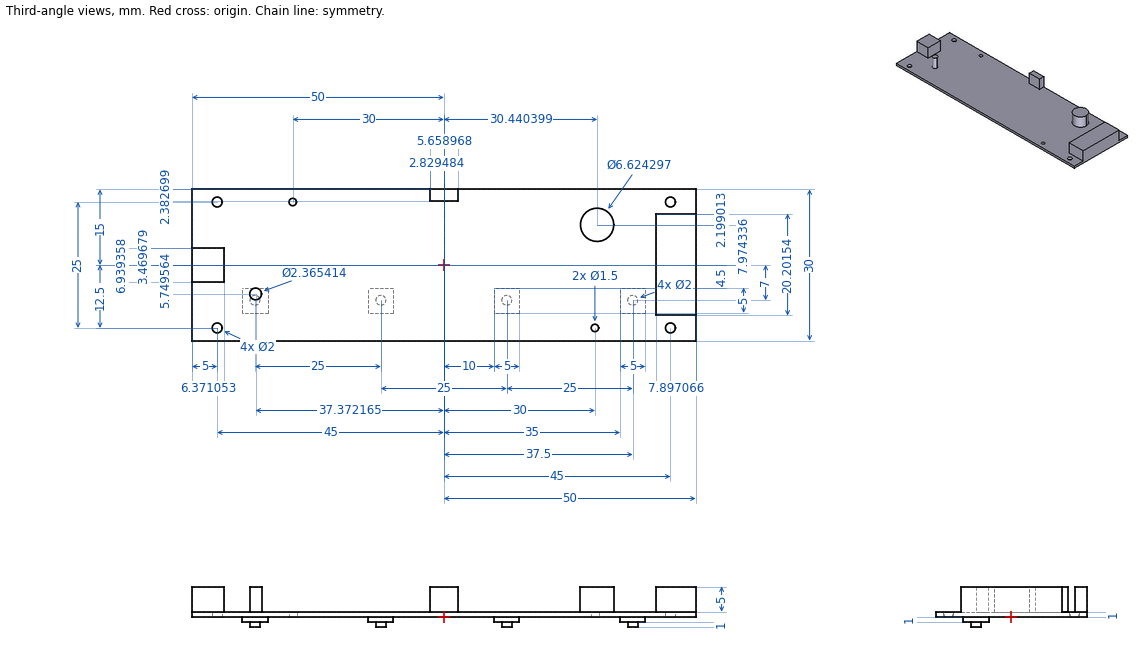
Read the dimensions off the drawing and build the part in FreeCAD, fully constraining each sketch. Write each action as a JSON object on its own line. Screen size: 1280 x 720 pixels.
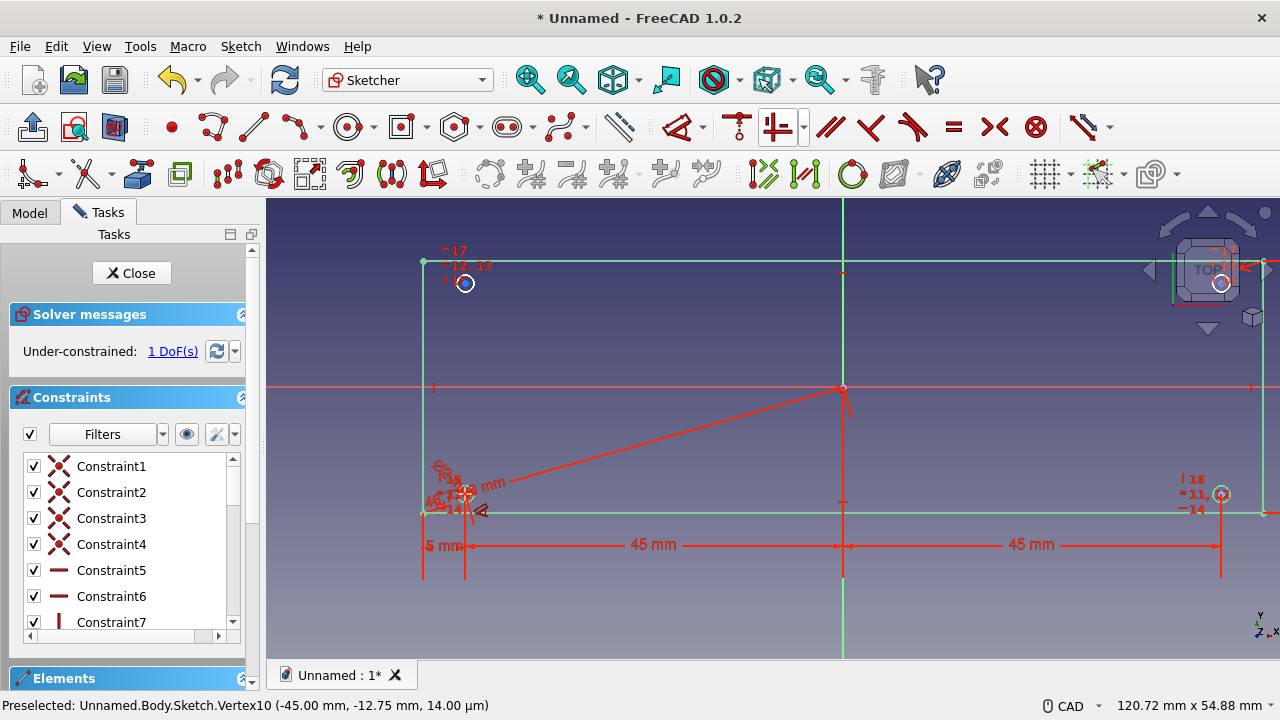
{"action": "left_click", "coordinate": [465, 284]}
{"action": "left_click", "coordinate": [499, 340]}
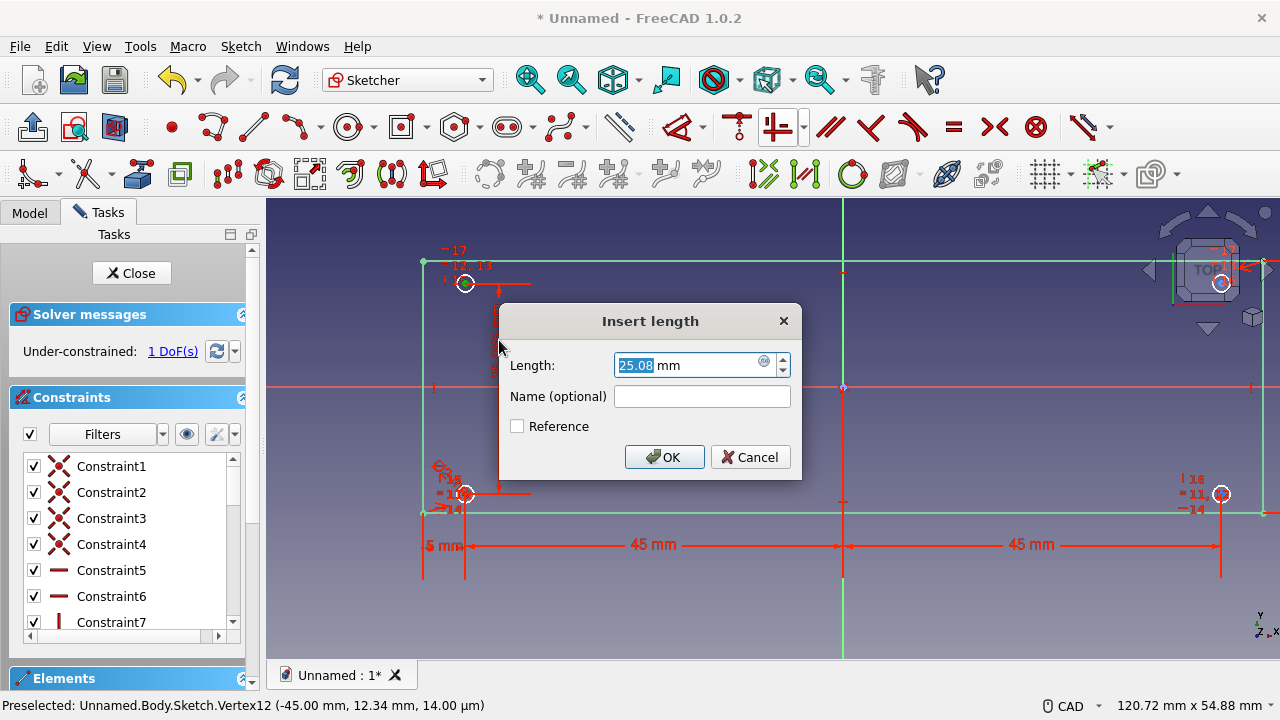
{"action": "type", "text": "25"}
{"action": "key", "text": "Return"}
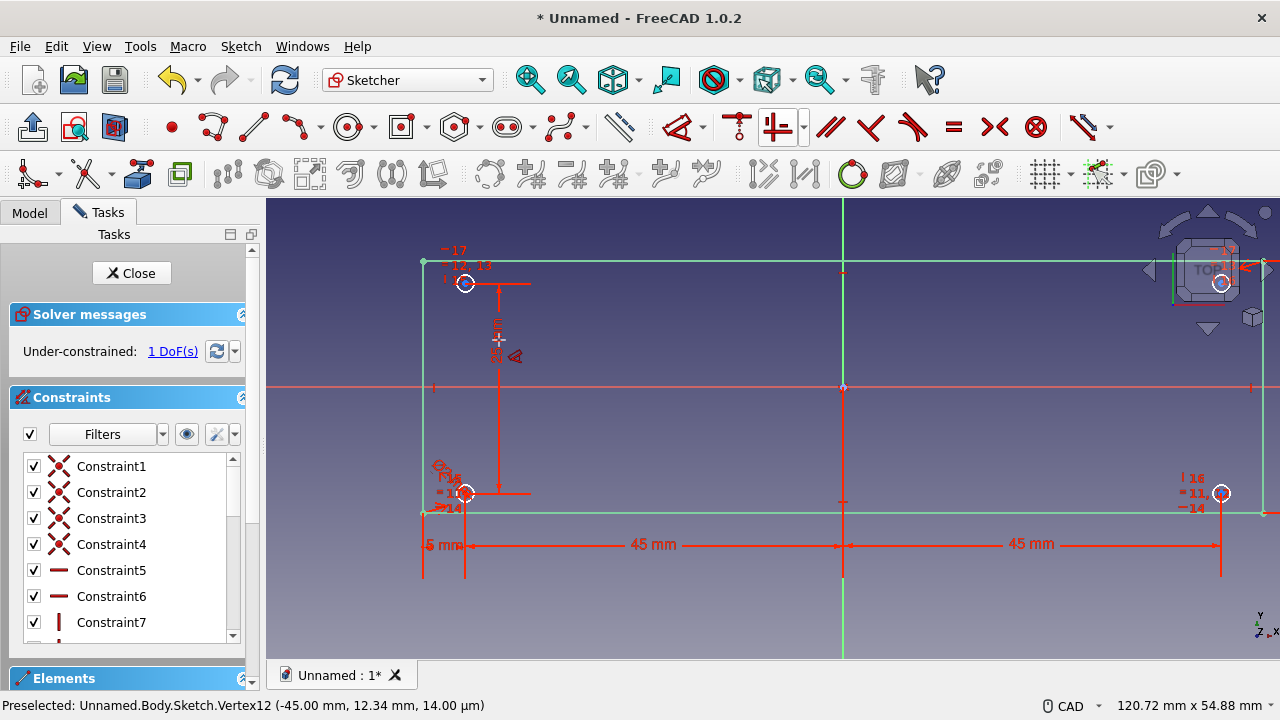
{"action": "left_click", "coordinate": [465, 494]}
{"action": "left_click", "coordinate": [877, 440]}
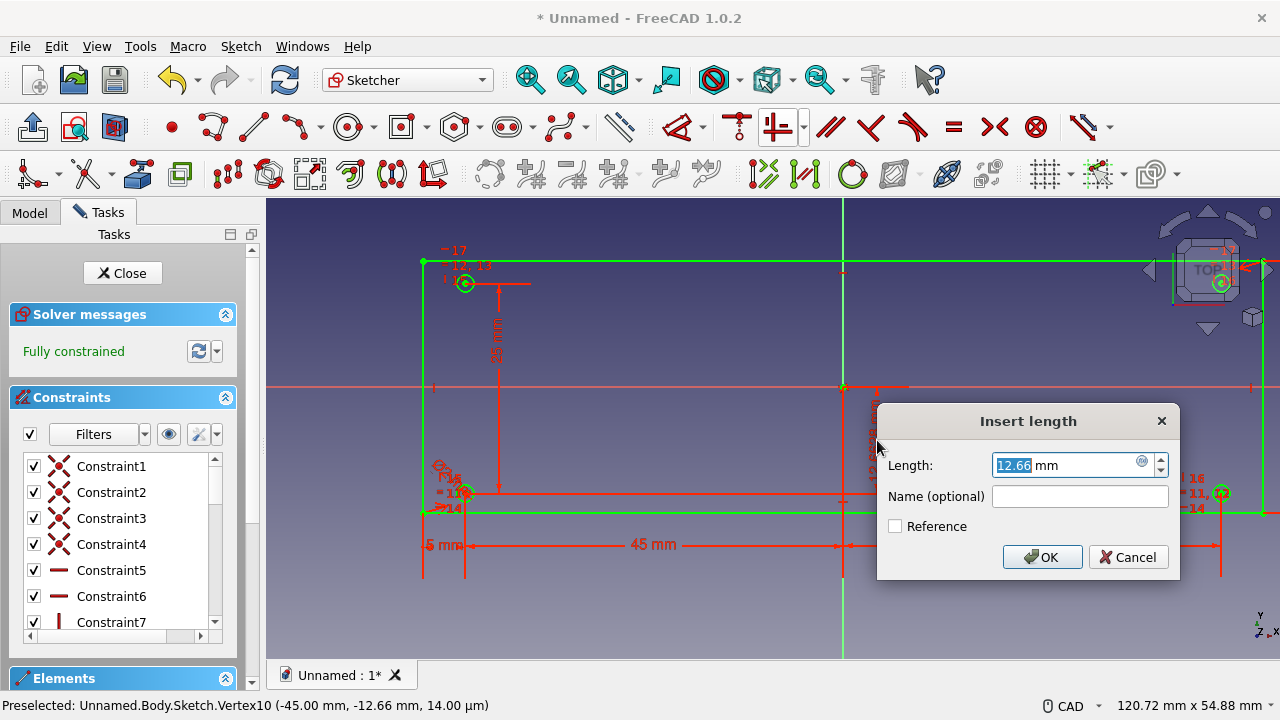
{"action": "type", "text": "12.5"}
{"action": "key", "text": "Return"}
{"action": "key", "text": "Escape"}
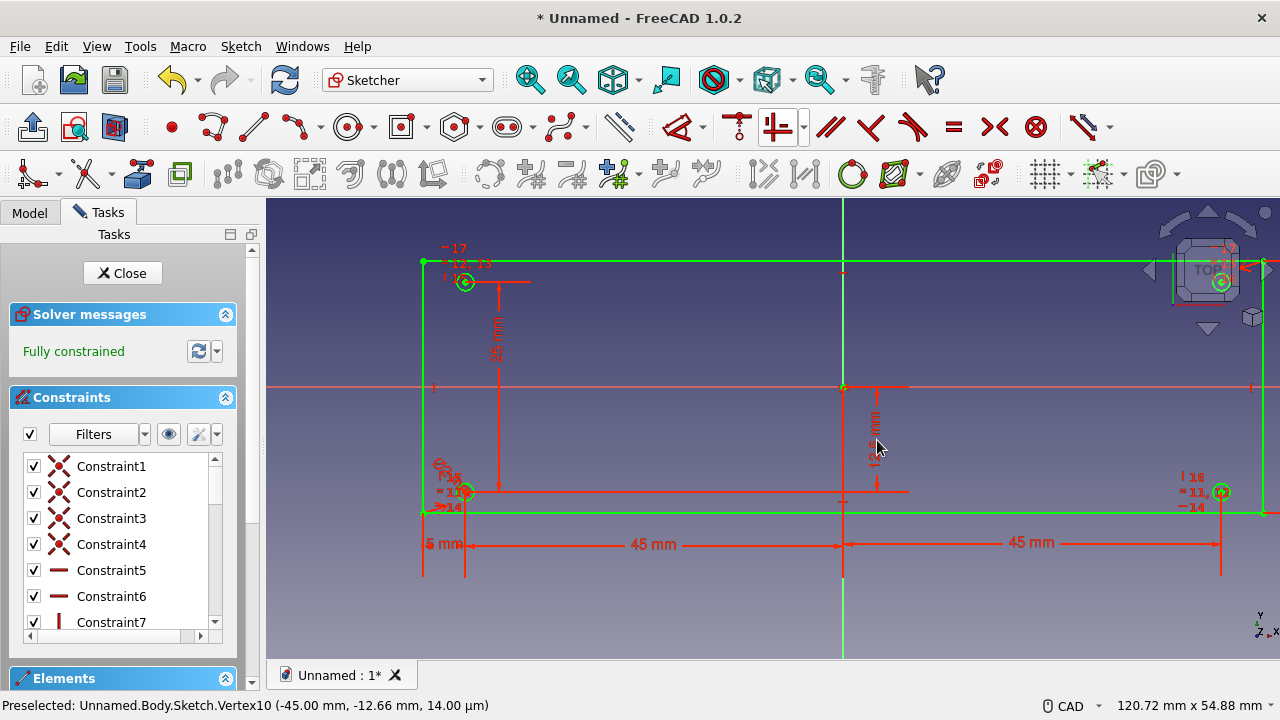
{"action": "left_click", "coordinate": [123, 273]}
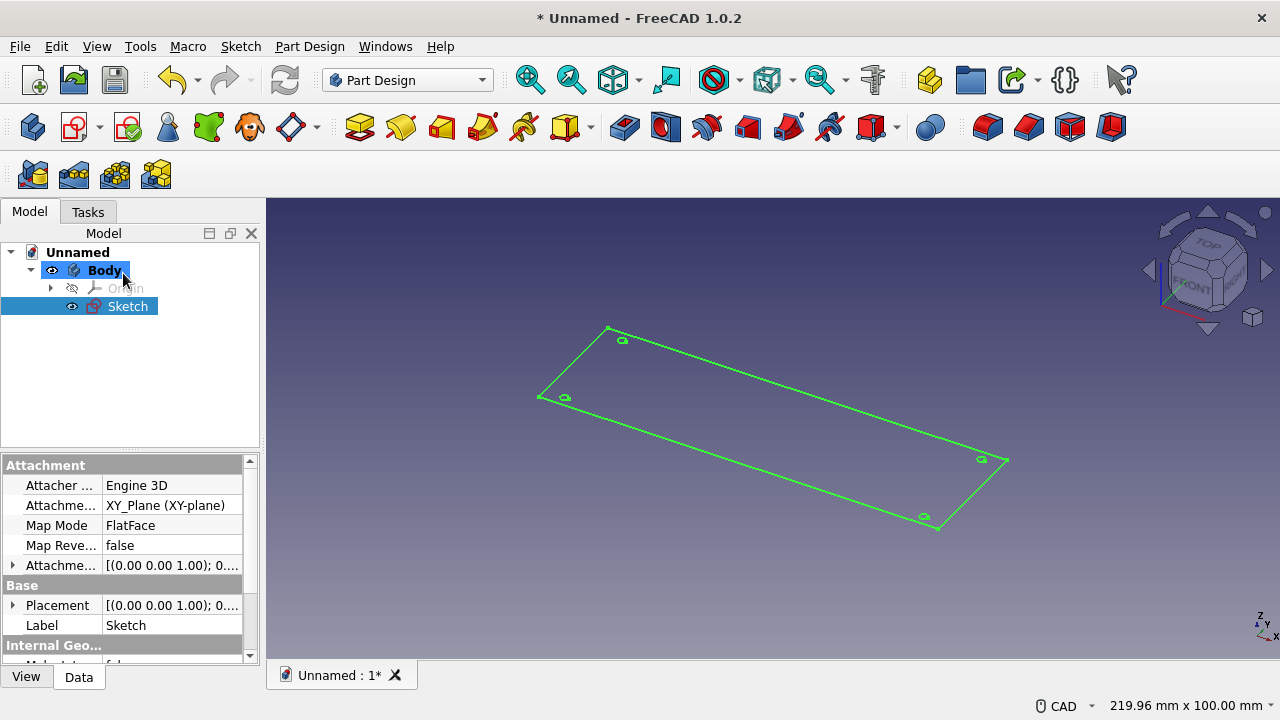
{"action": "left_click", "coordinate": [360, 128]}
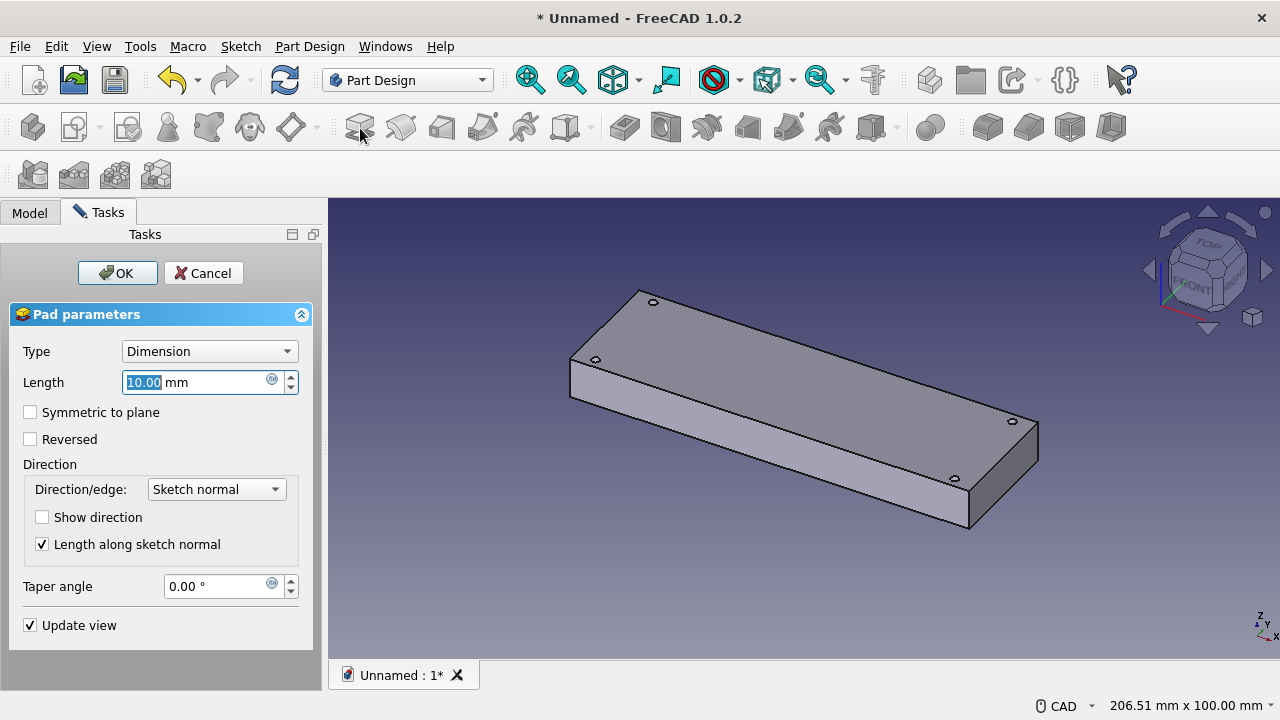
{"action": "type", "text": "1"}
{"action": "key", "text": "Tab"}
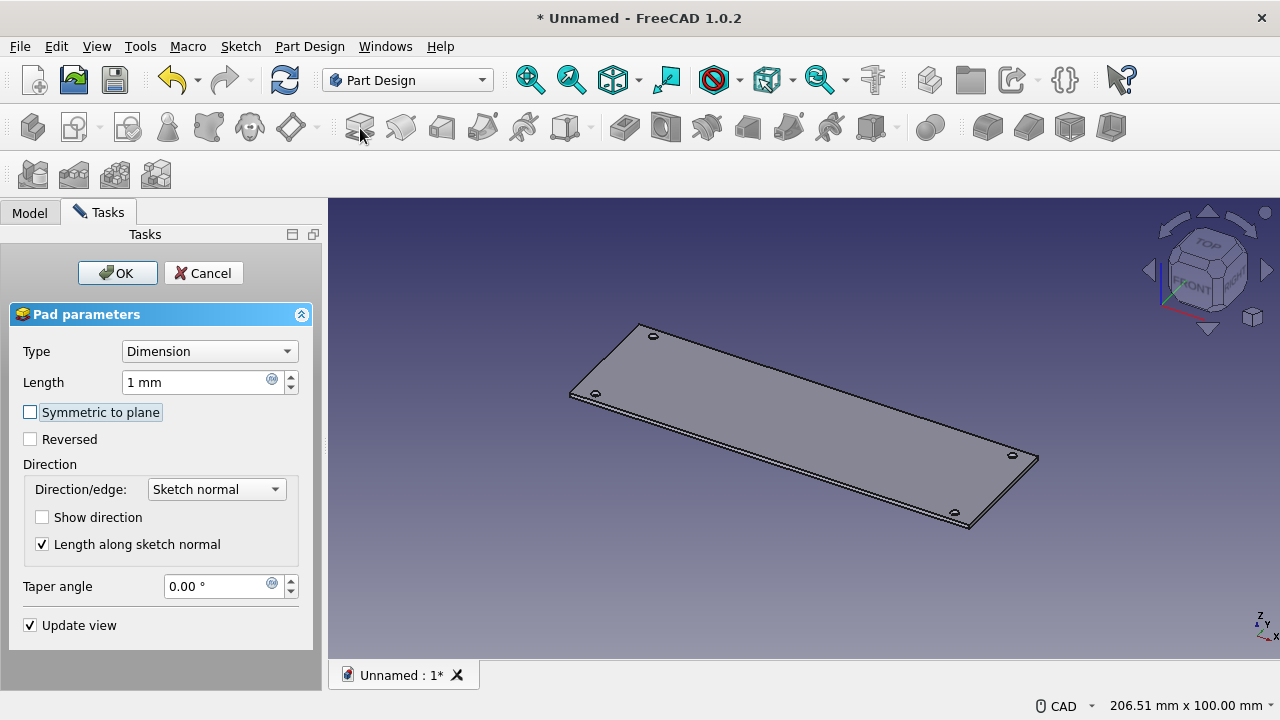
{"action": "left_click", "coordinate": [118, 273]}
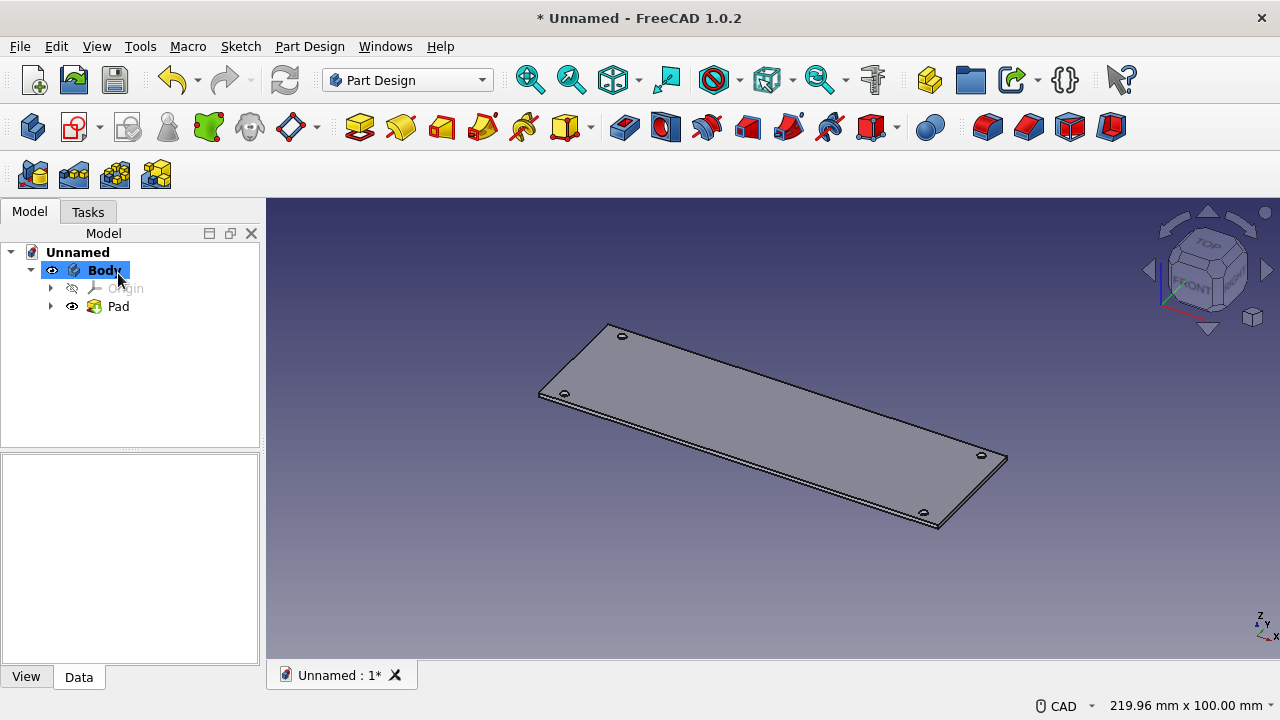
{"action": "left_click", "coordinate": [887, 461]}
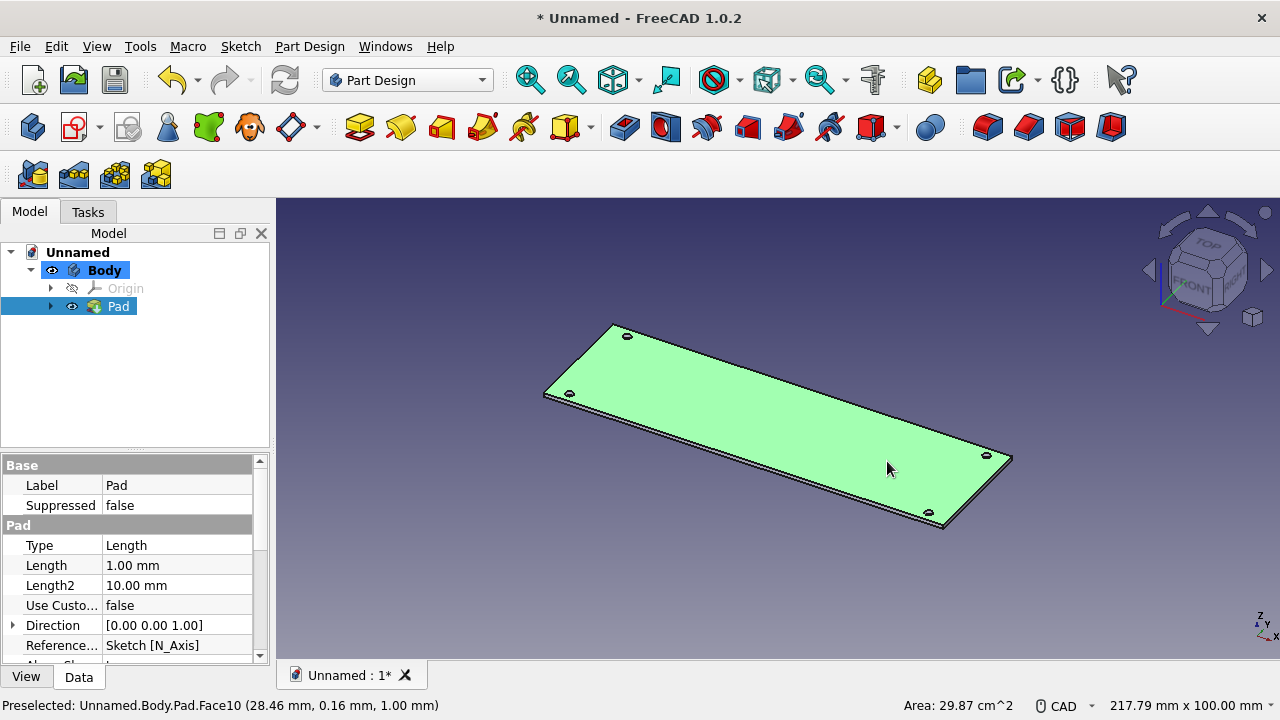
{"action": "left_click", "coordinate": [74, 128]}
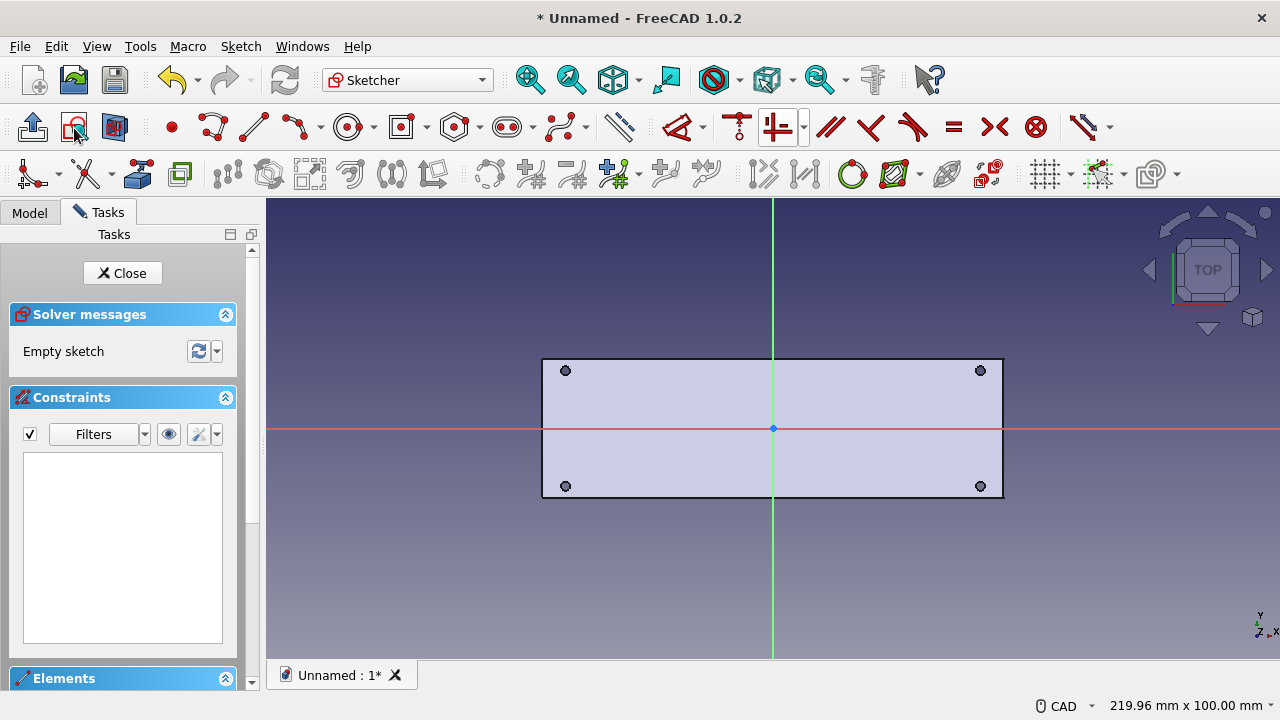
{"action": "key", "text": "g r"}